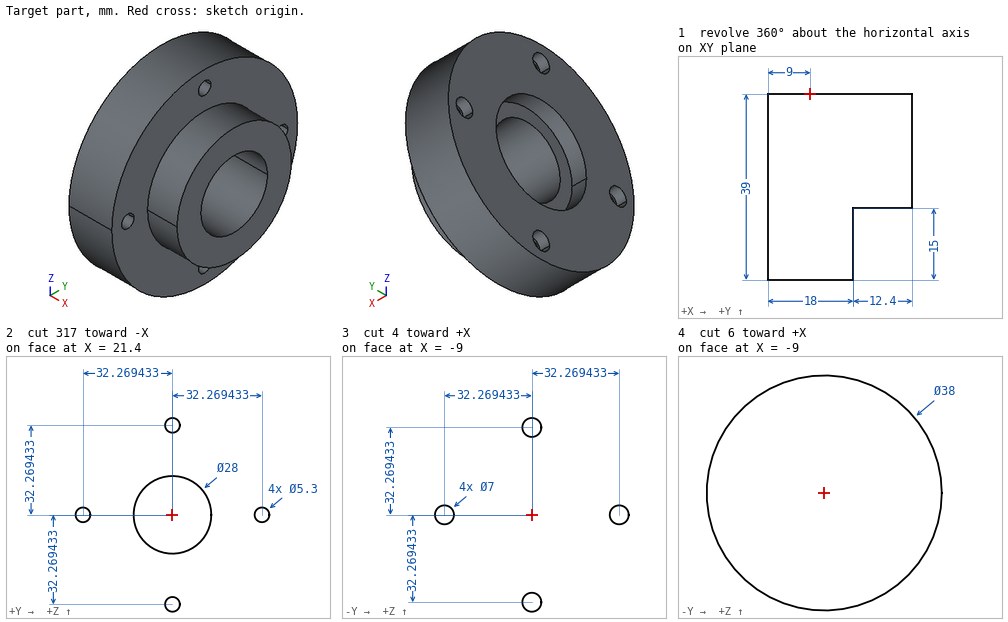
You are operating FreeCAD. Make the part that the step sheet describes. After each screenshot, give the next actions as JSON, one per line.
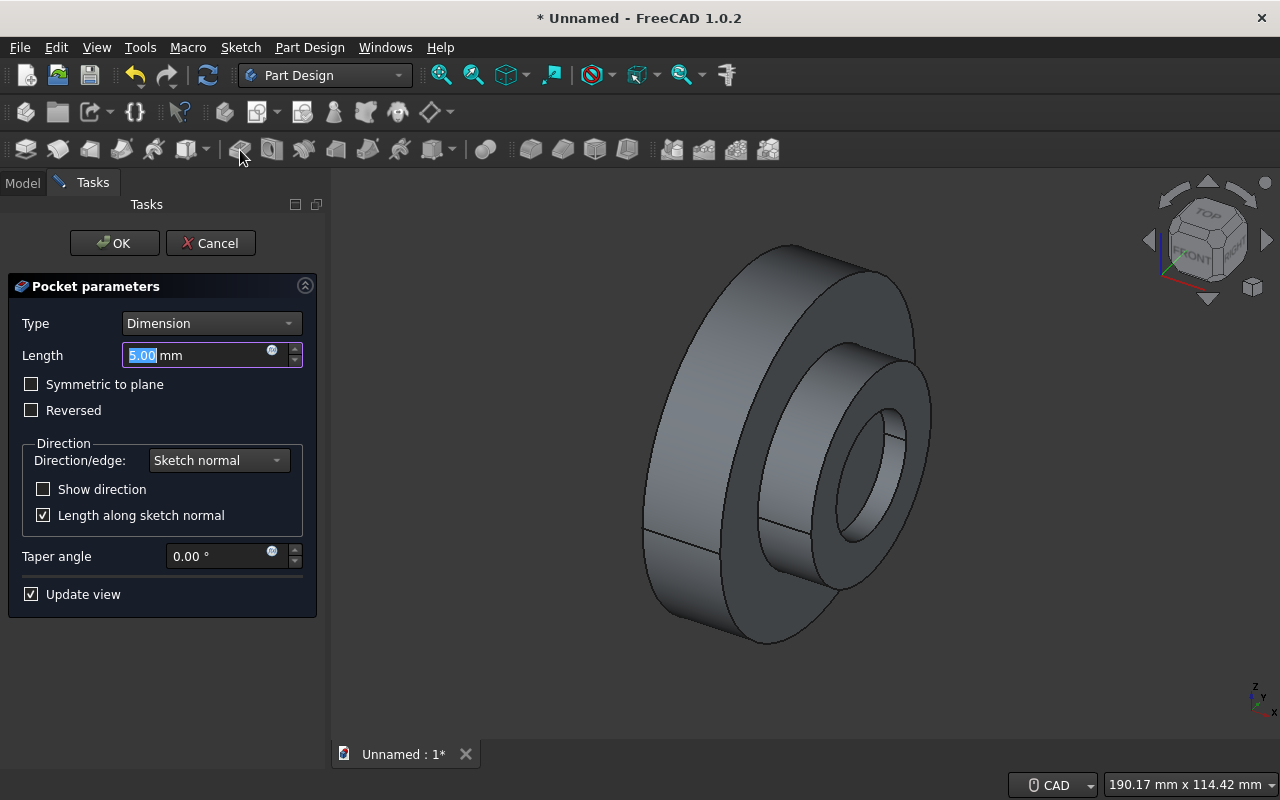
{"action": "type", "text": "317"}
{"action": "key", "text": "Tab"}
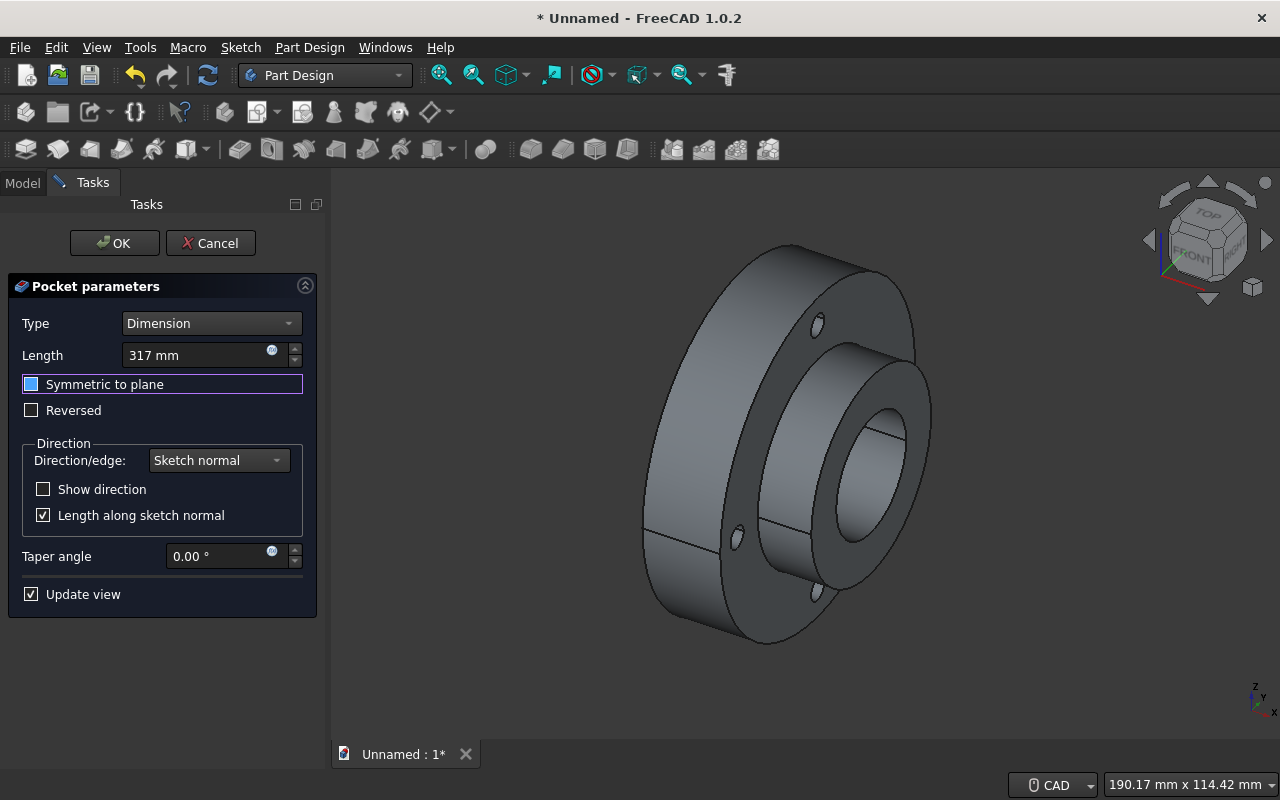
{"action": "left_click", "coordinate": [115, 243]}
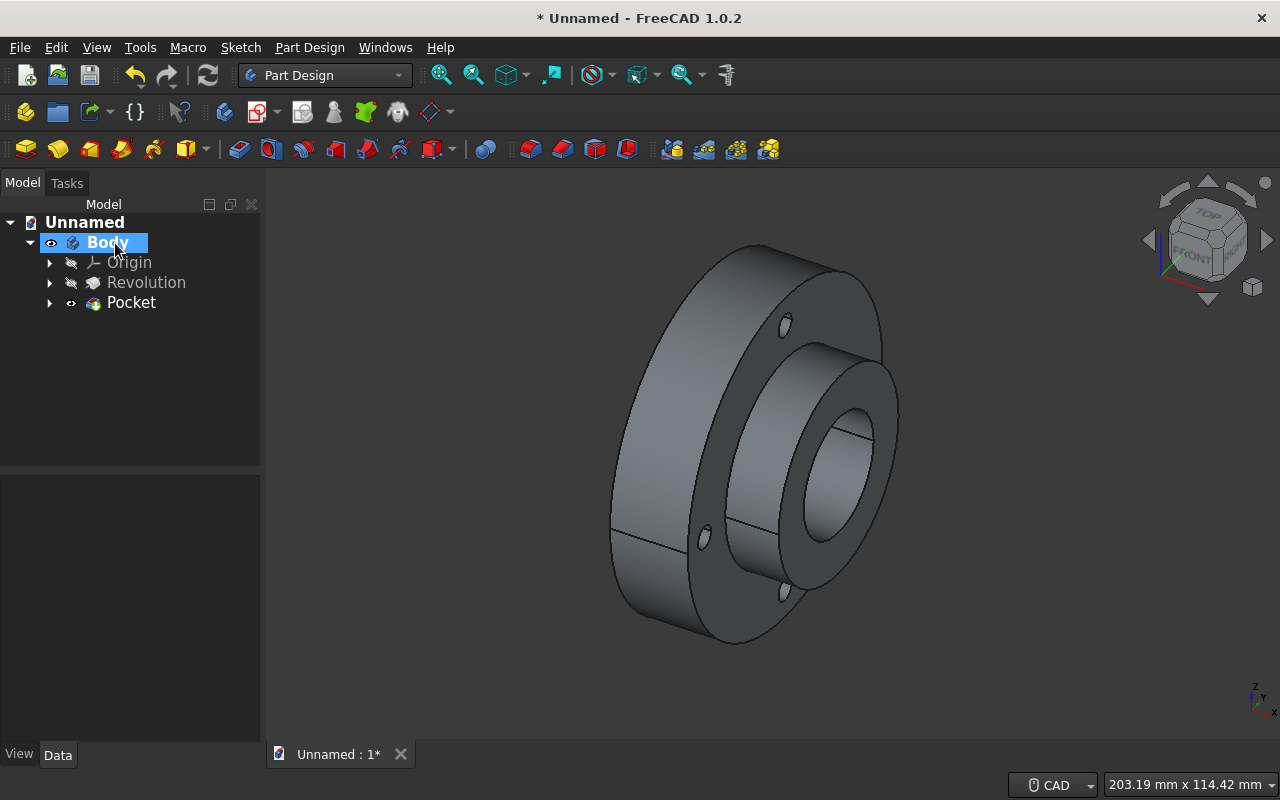
{"action": "key", "text": "6"}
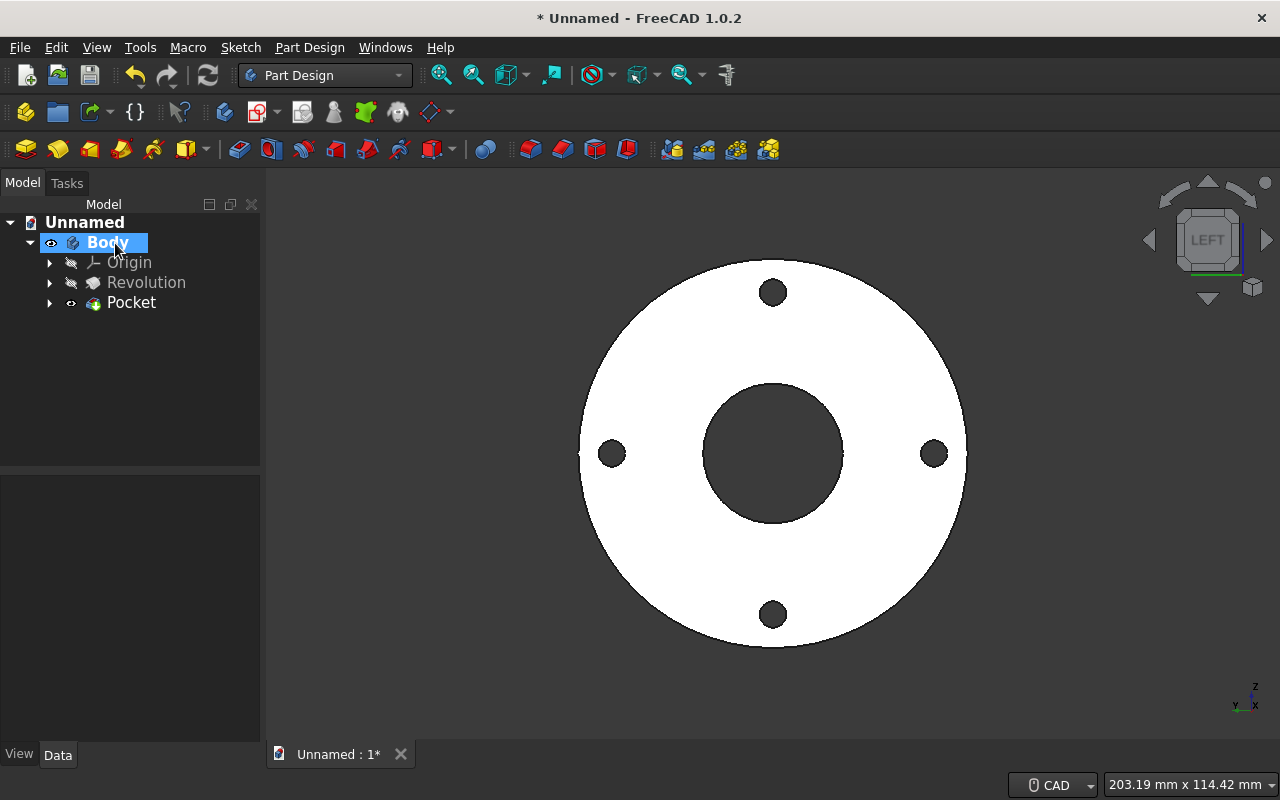
{"action": "left_click", "coordinate": [662, 397]}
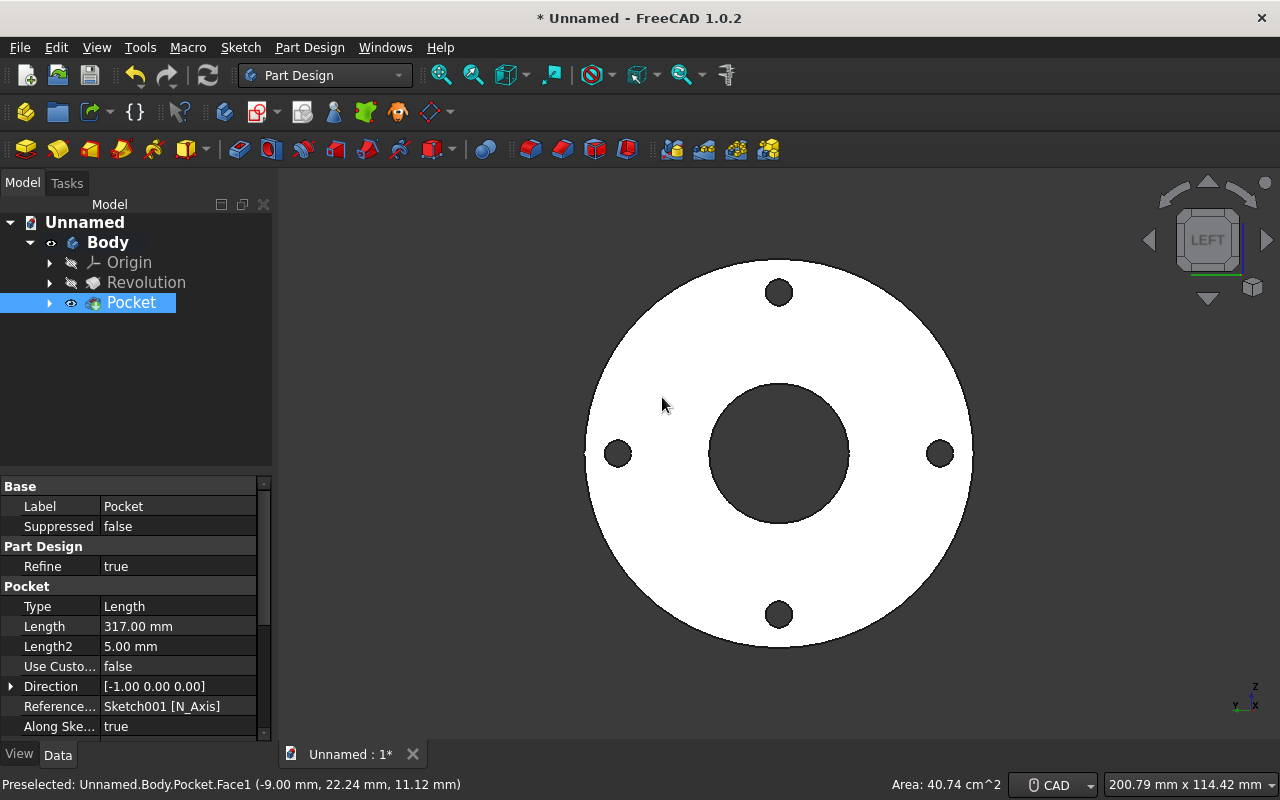
{"action": "left_click", "coordinate": [258, 112]}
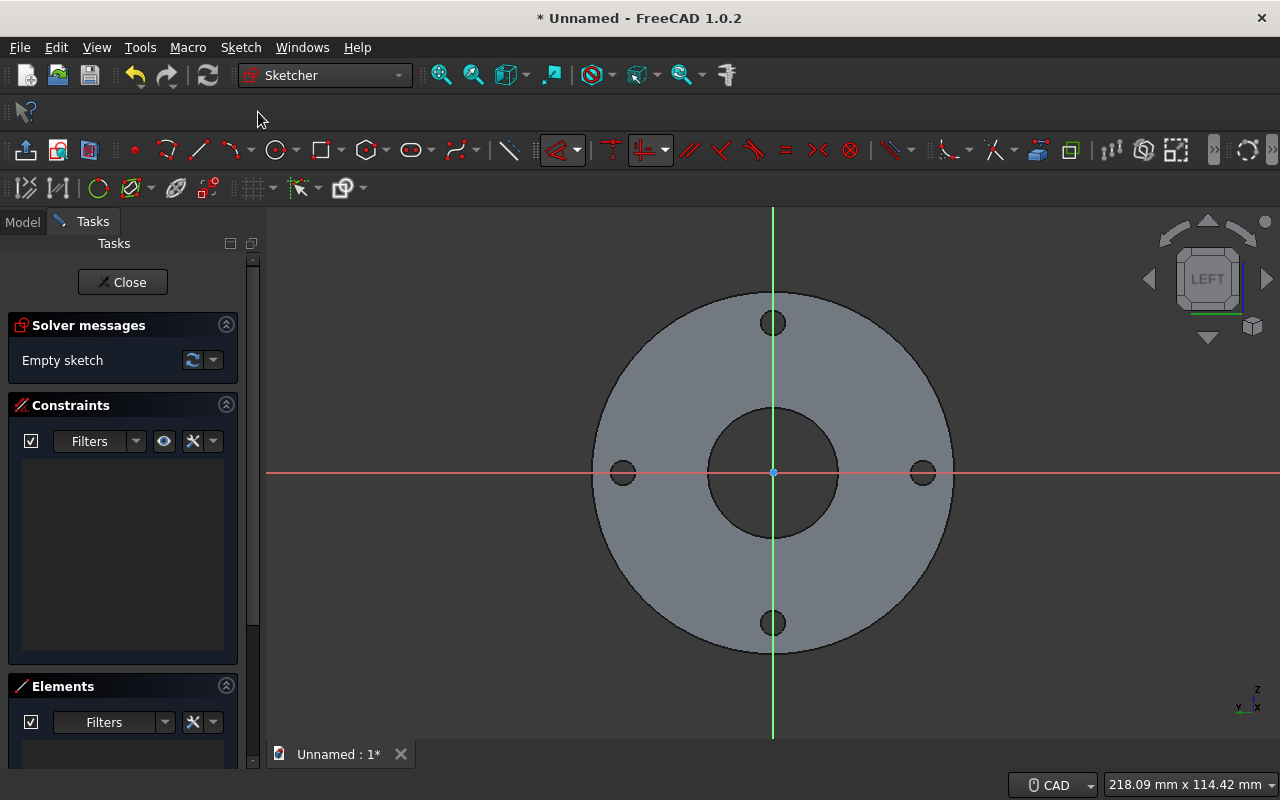
{"action": "left_click", "coordinate": [276, 150]}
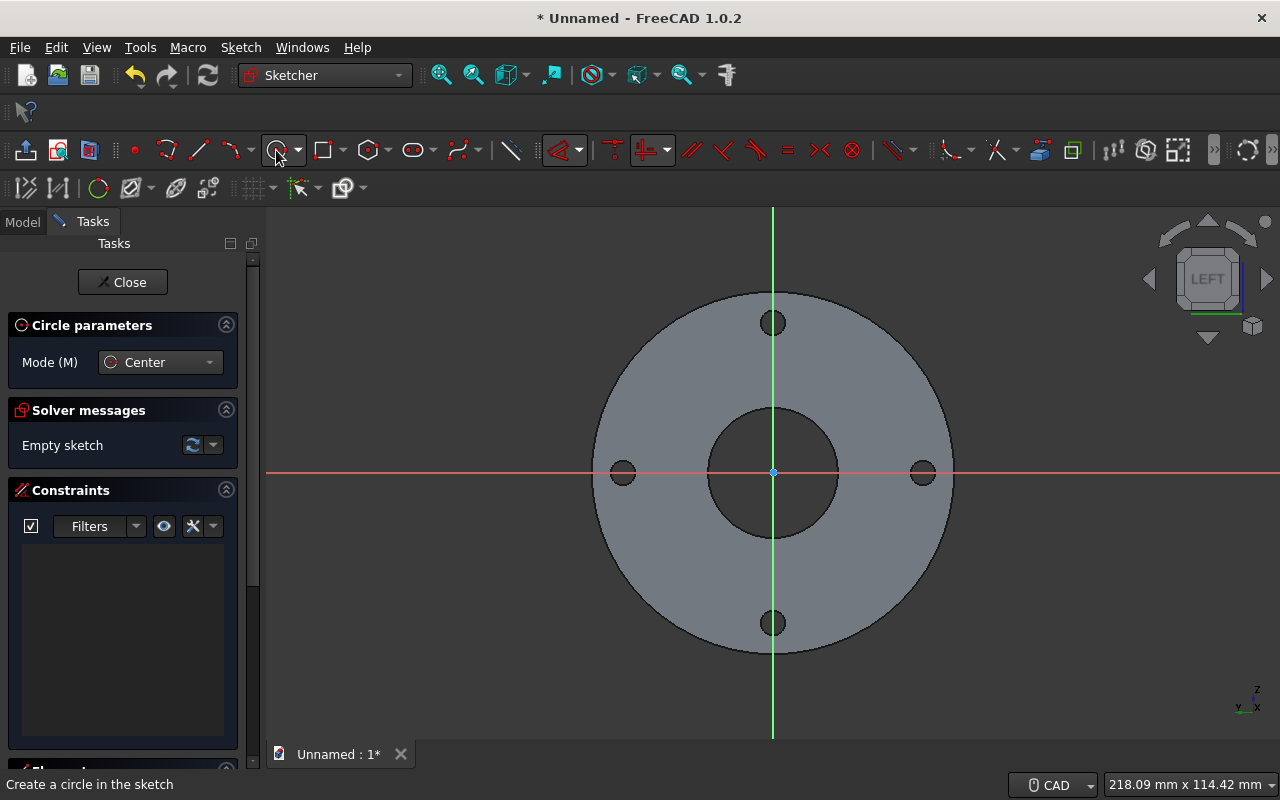
{"action": "scroll", "coordinate": [623, 473], "scroll_direction": "up", "scroll_amount": 2}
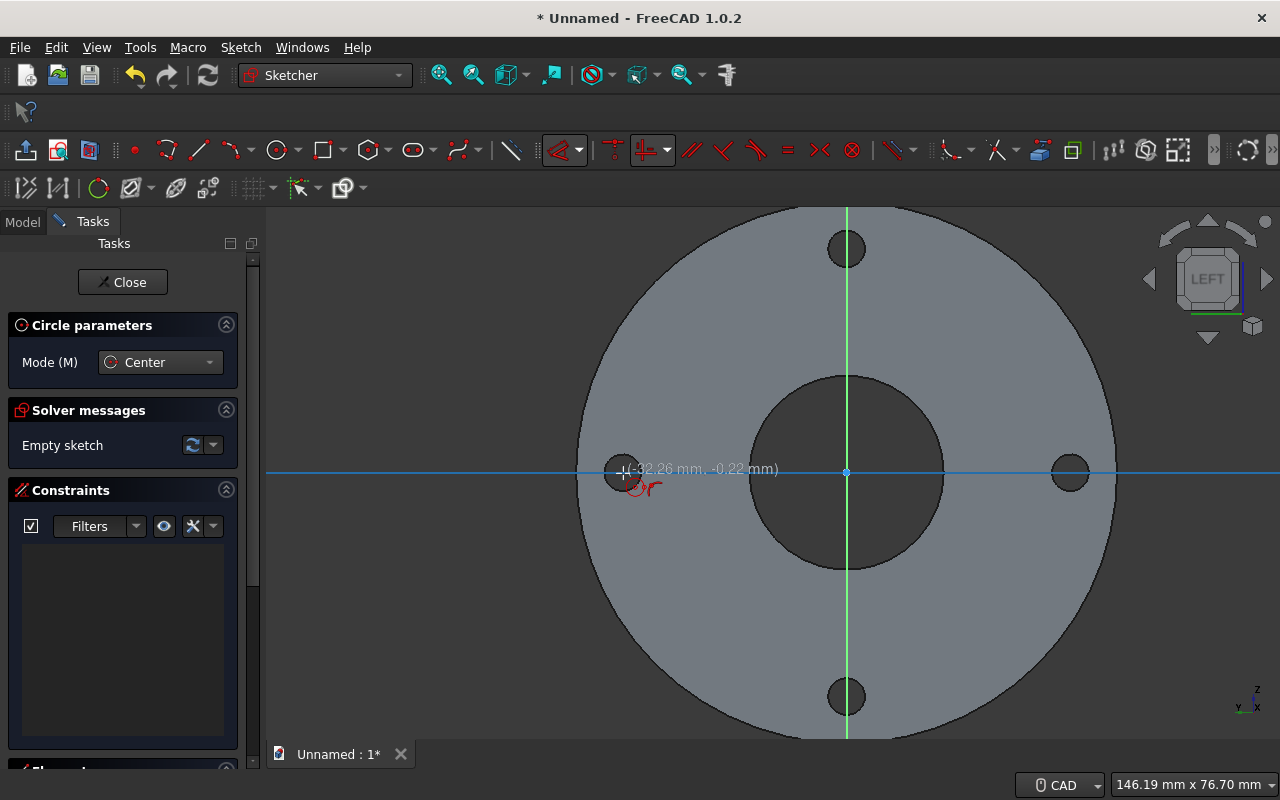
{"action": "left_click", "coordinate": [623, 473]}
{"action": "left_click", "coordinate": [640, 456]}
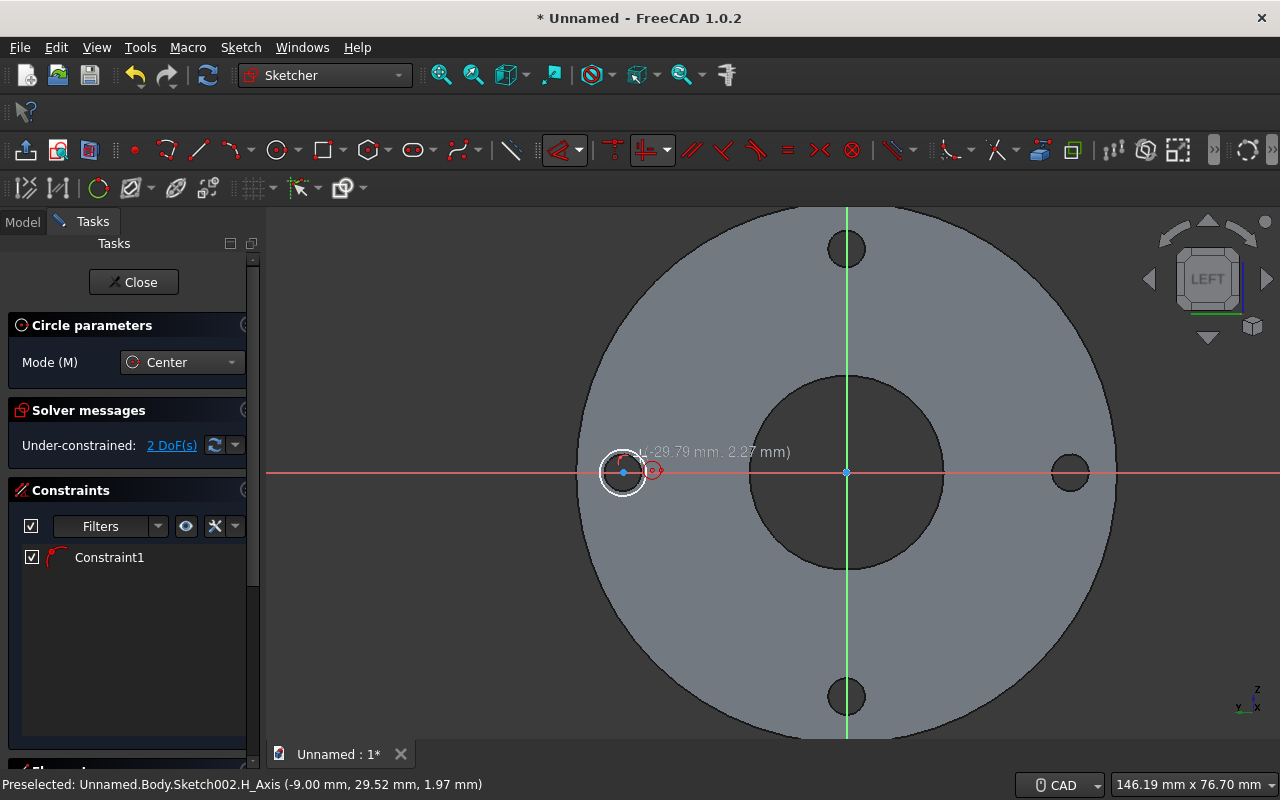
{"action": "left_click", "coordinate": [847, 697]}
{"action": "left_click", "coordinate": [864, 679]}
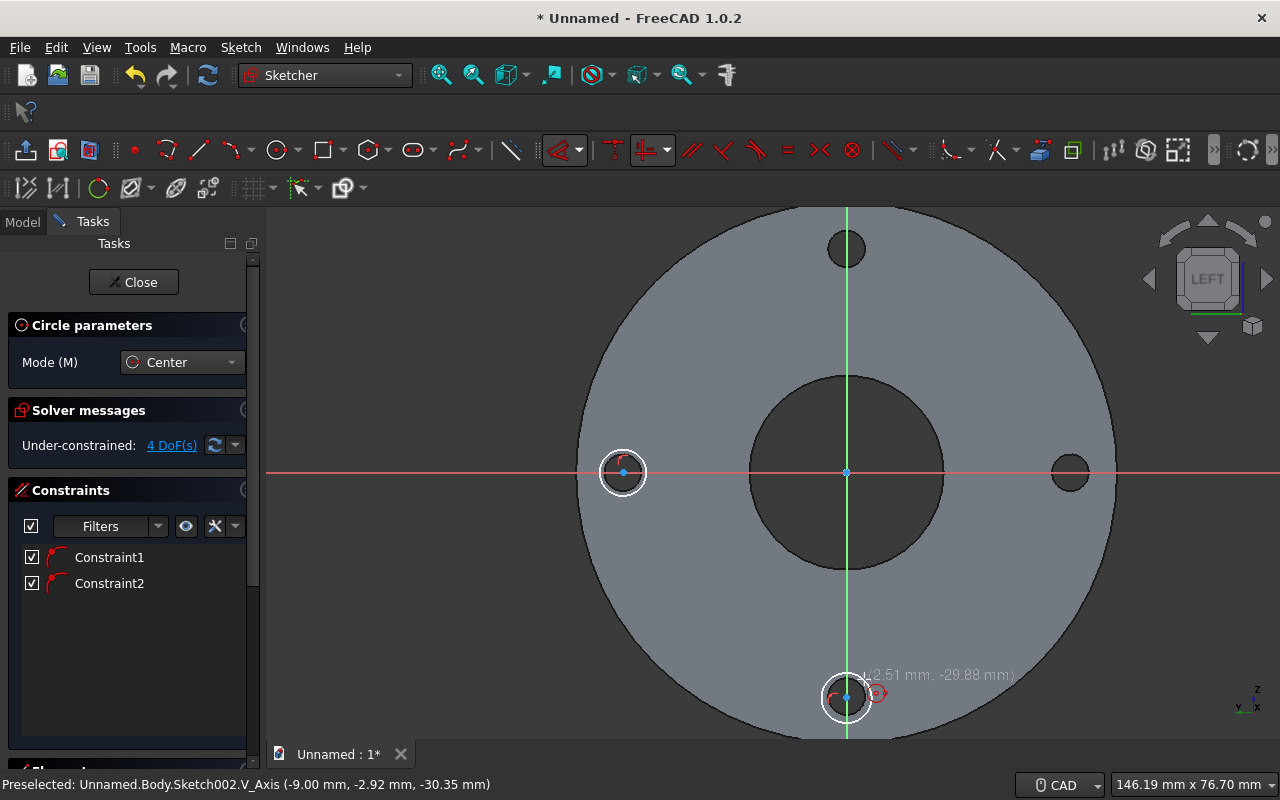
{"action": "left_click", "coordinate": [1070, 473]}
{"action": "left_click", "coordinate": [1088, 456]}